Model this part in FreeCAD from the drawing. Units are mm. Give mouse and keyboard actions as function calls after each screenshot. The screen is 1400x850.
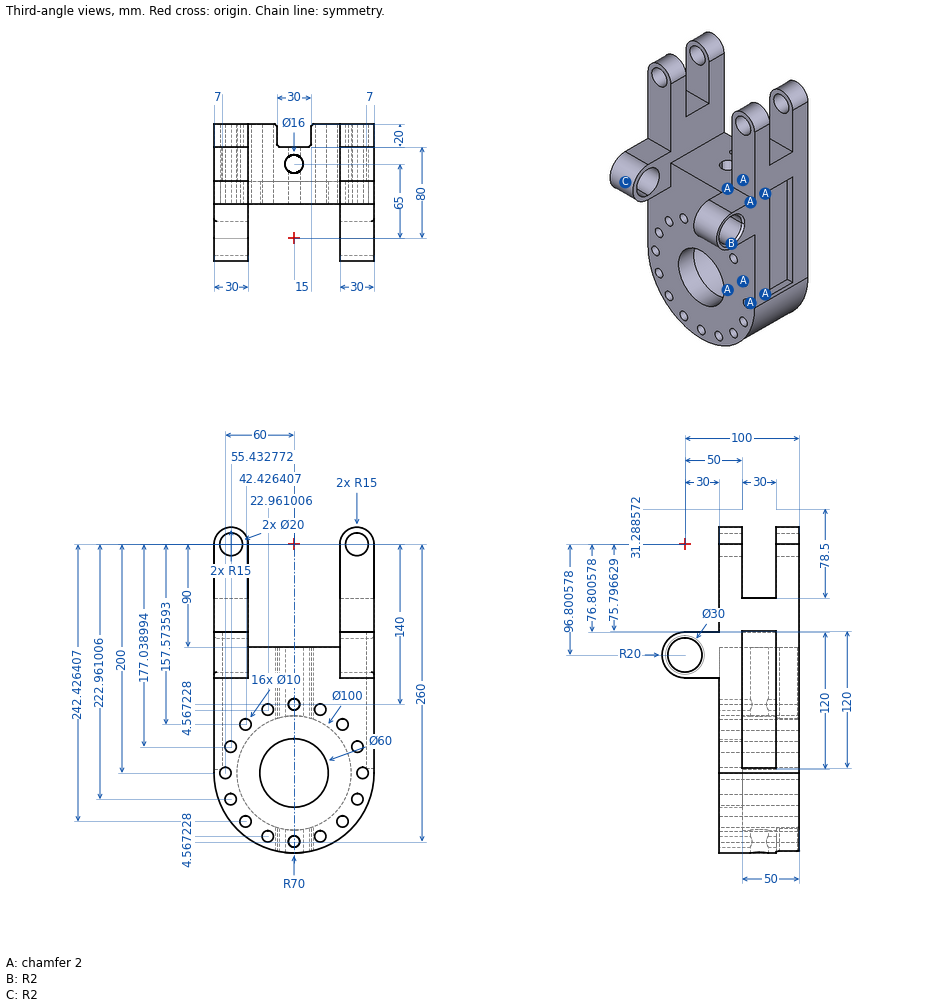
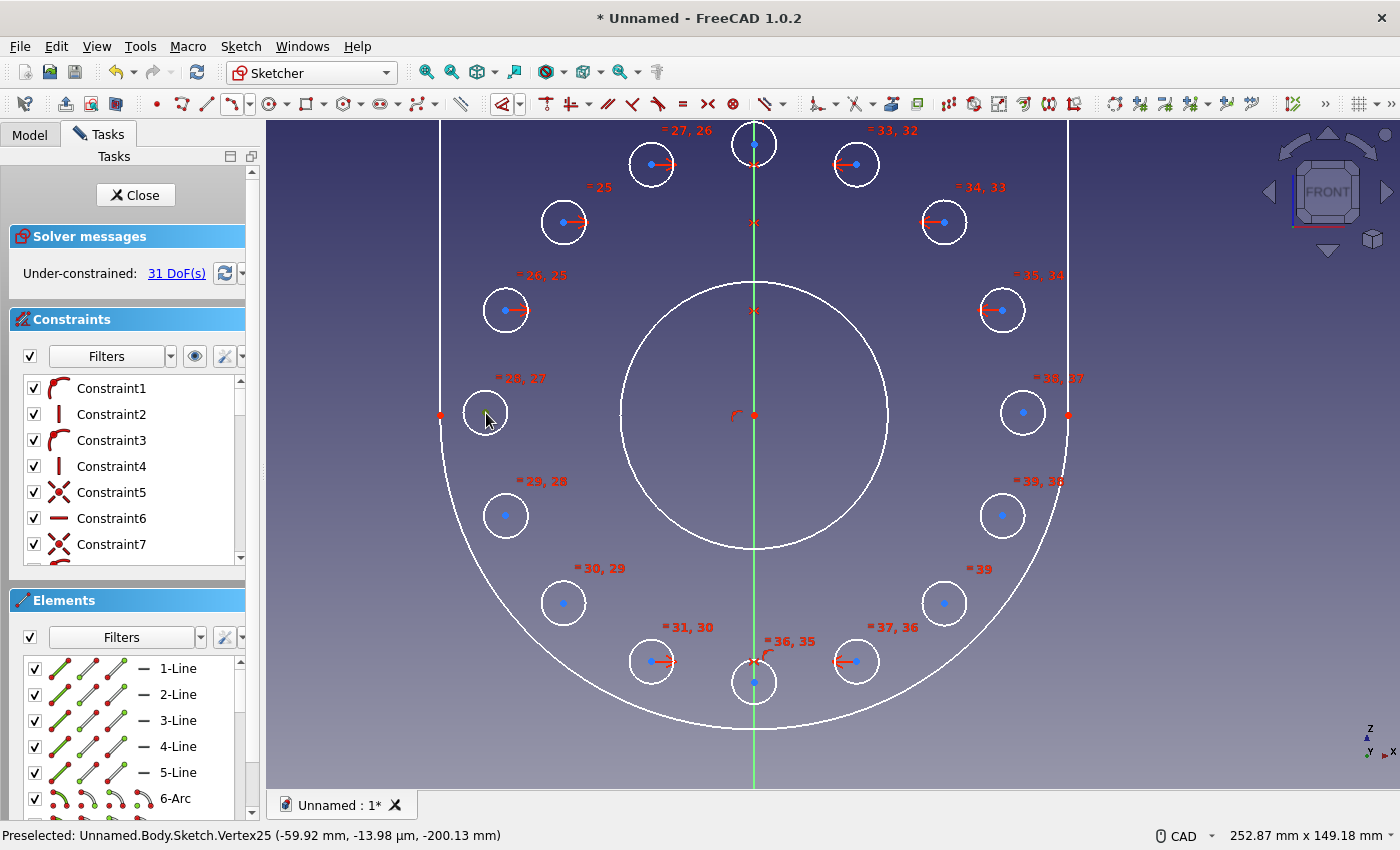
click(1023, 413)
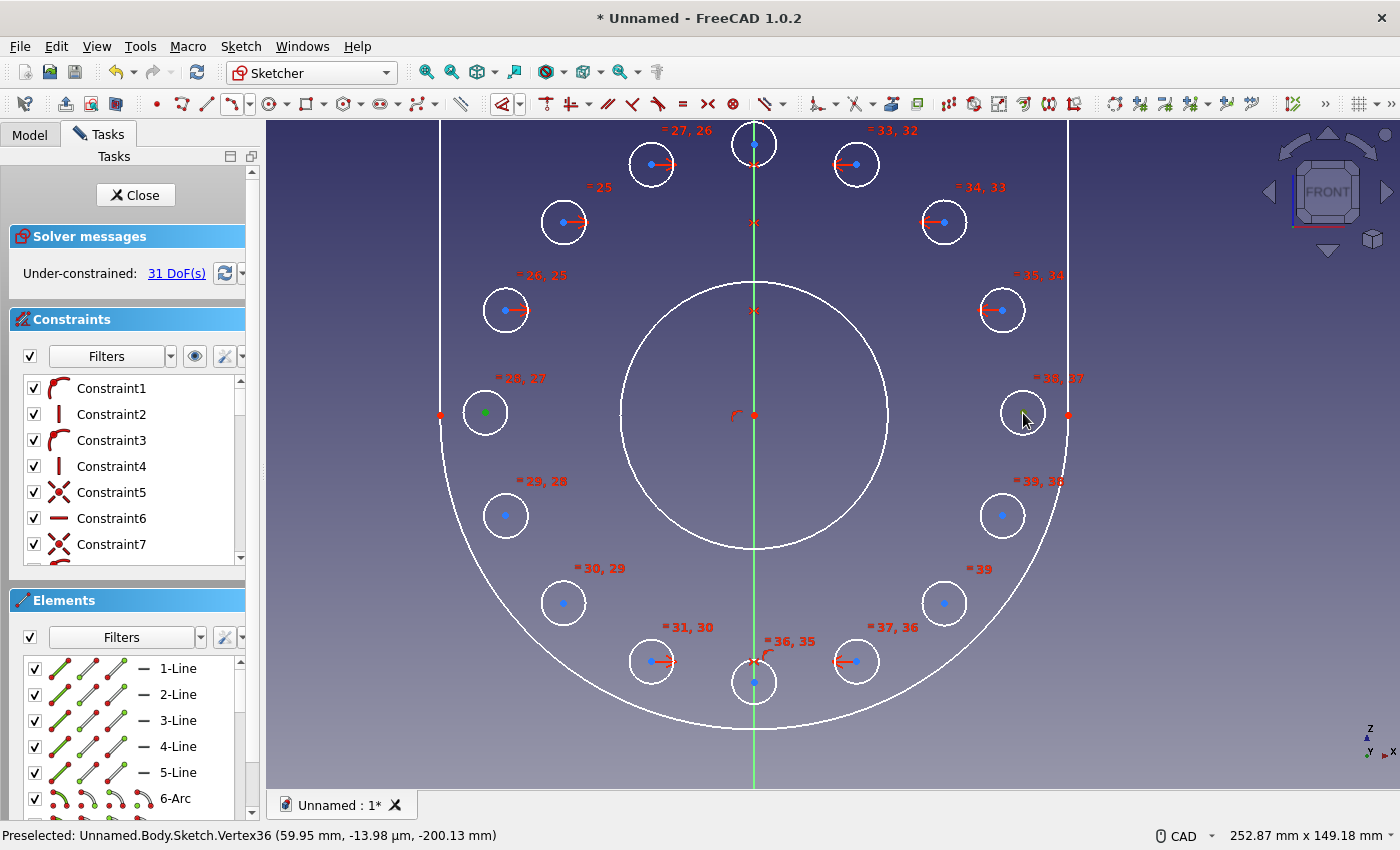
click(754, 630)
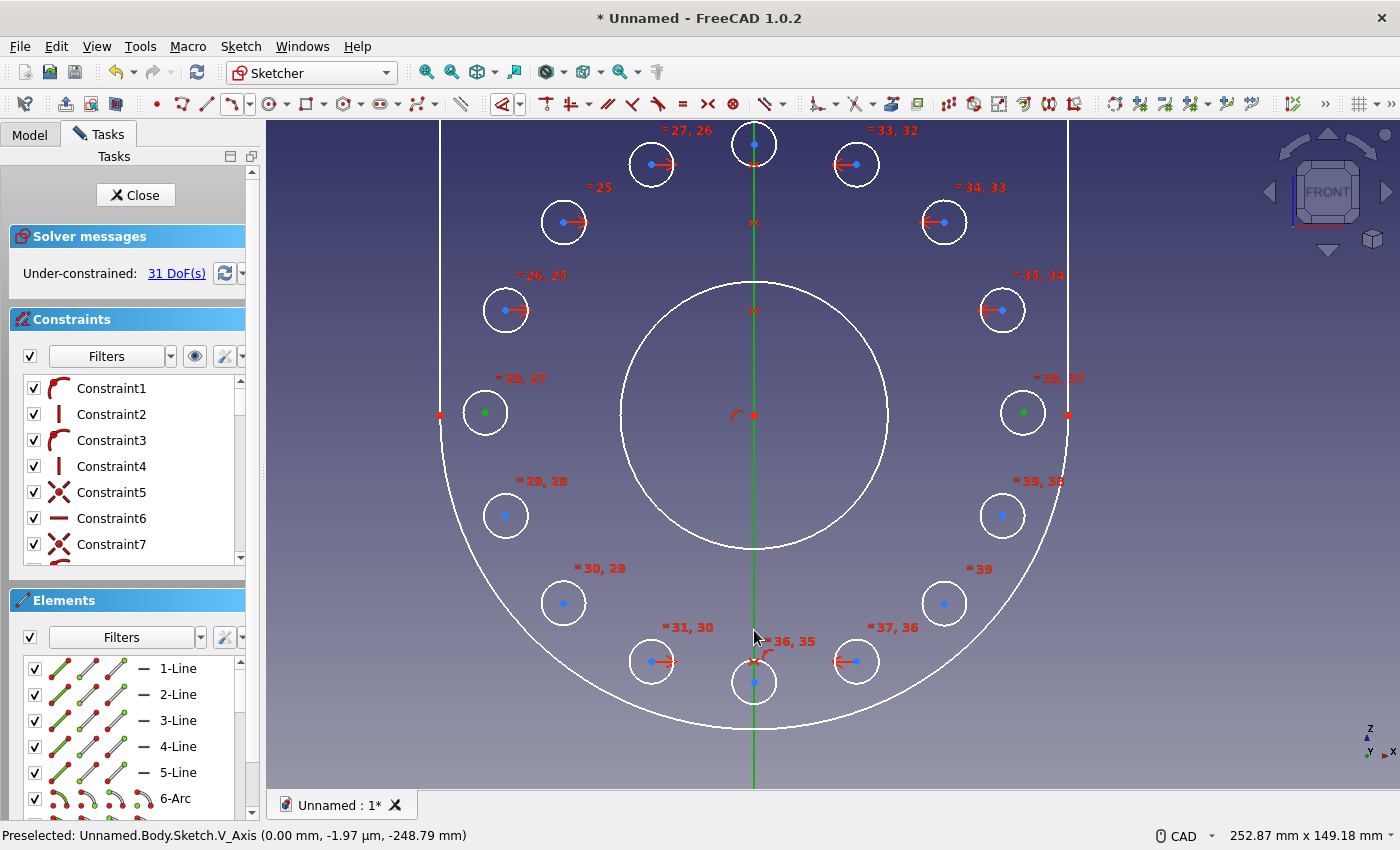
click(708, 104)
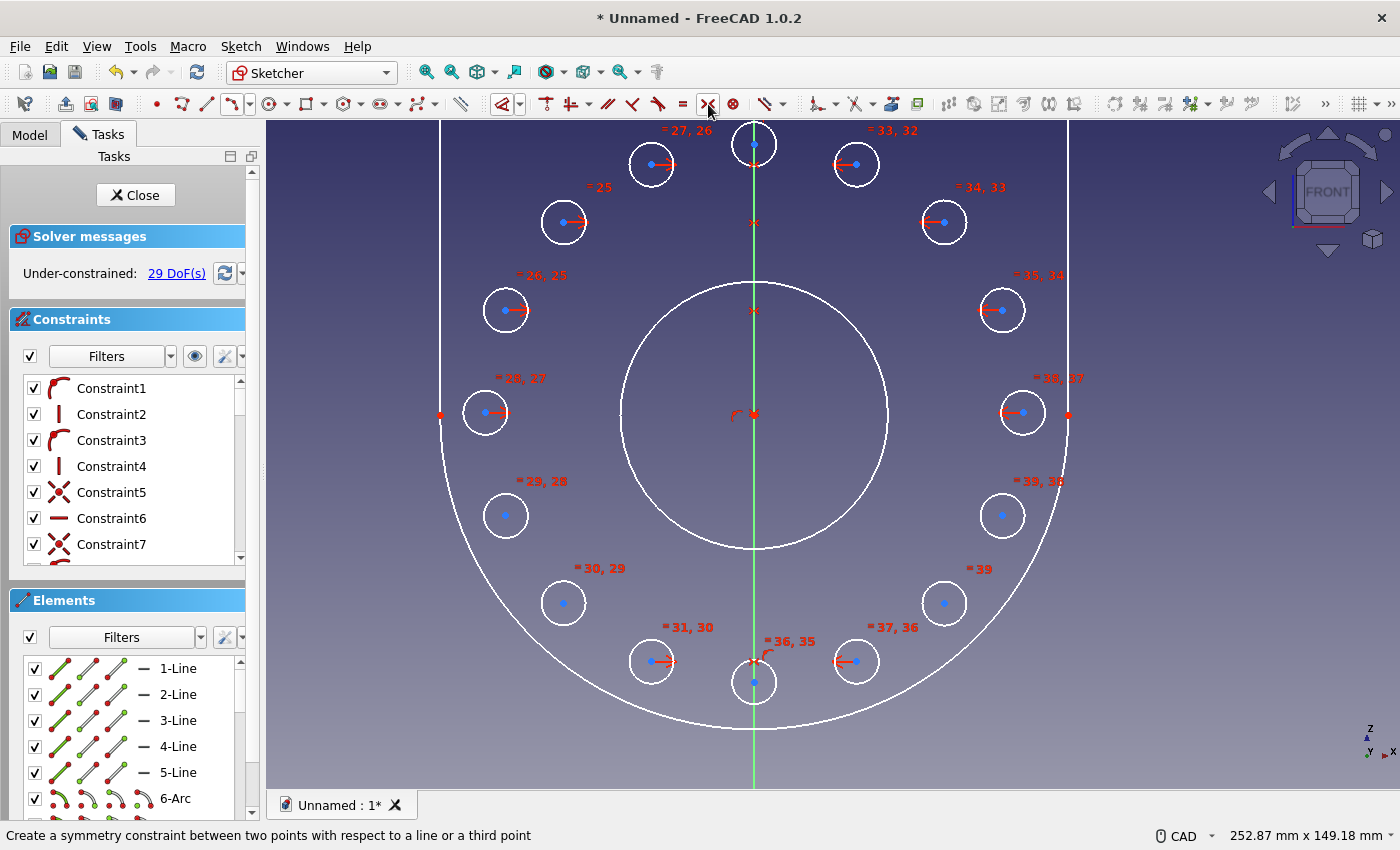
click(506, 516)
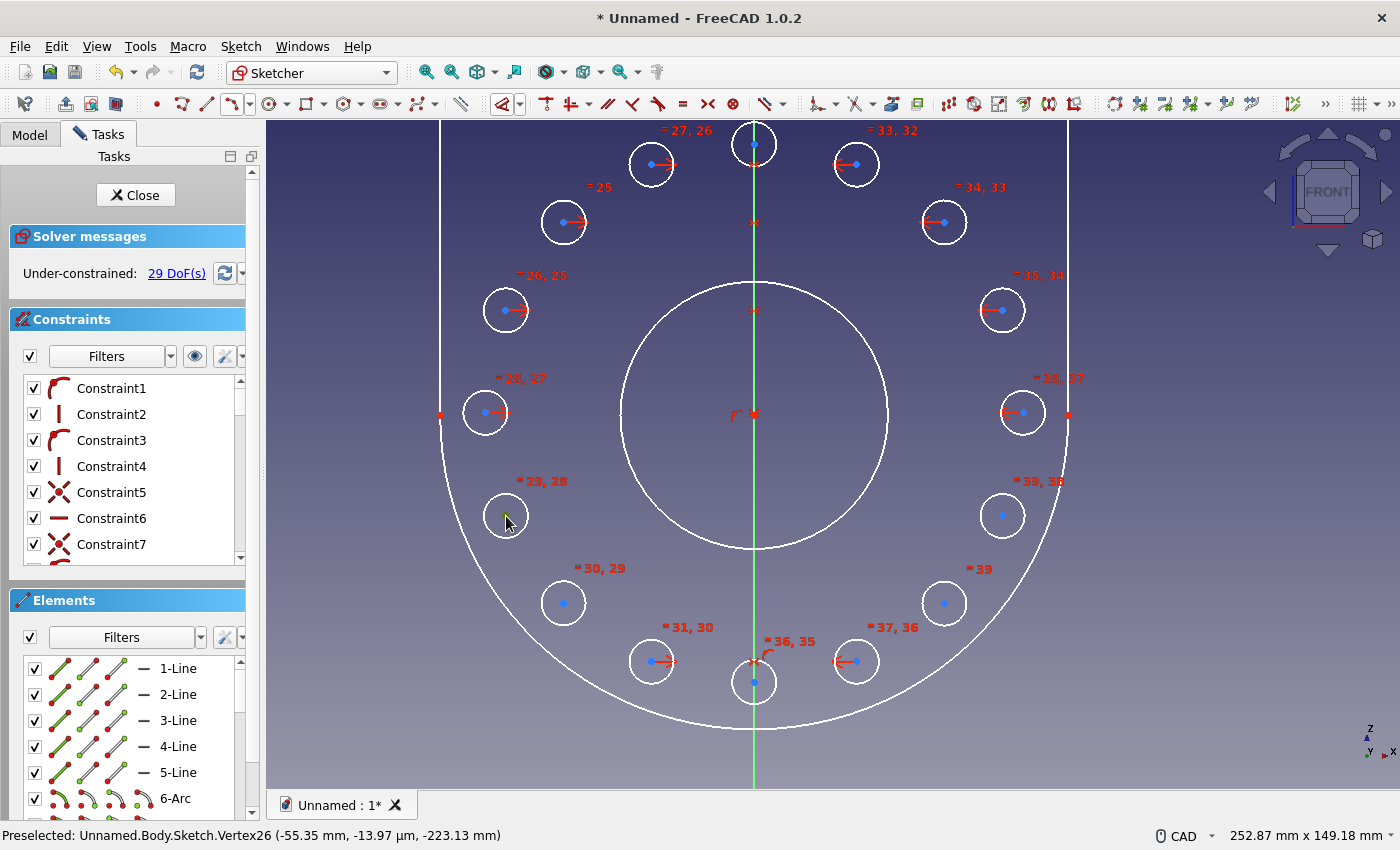
click(1003, 516)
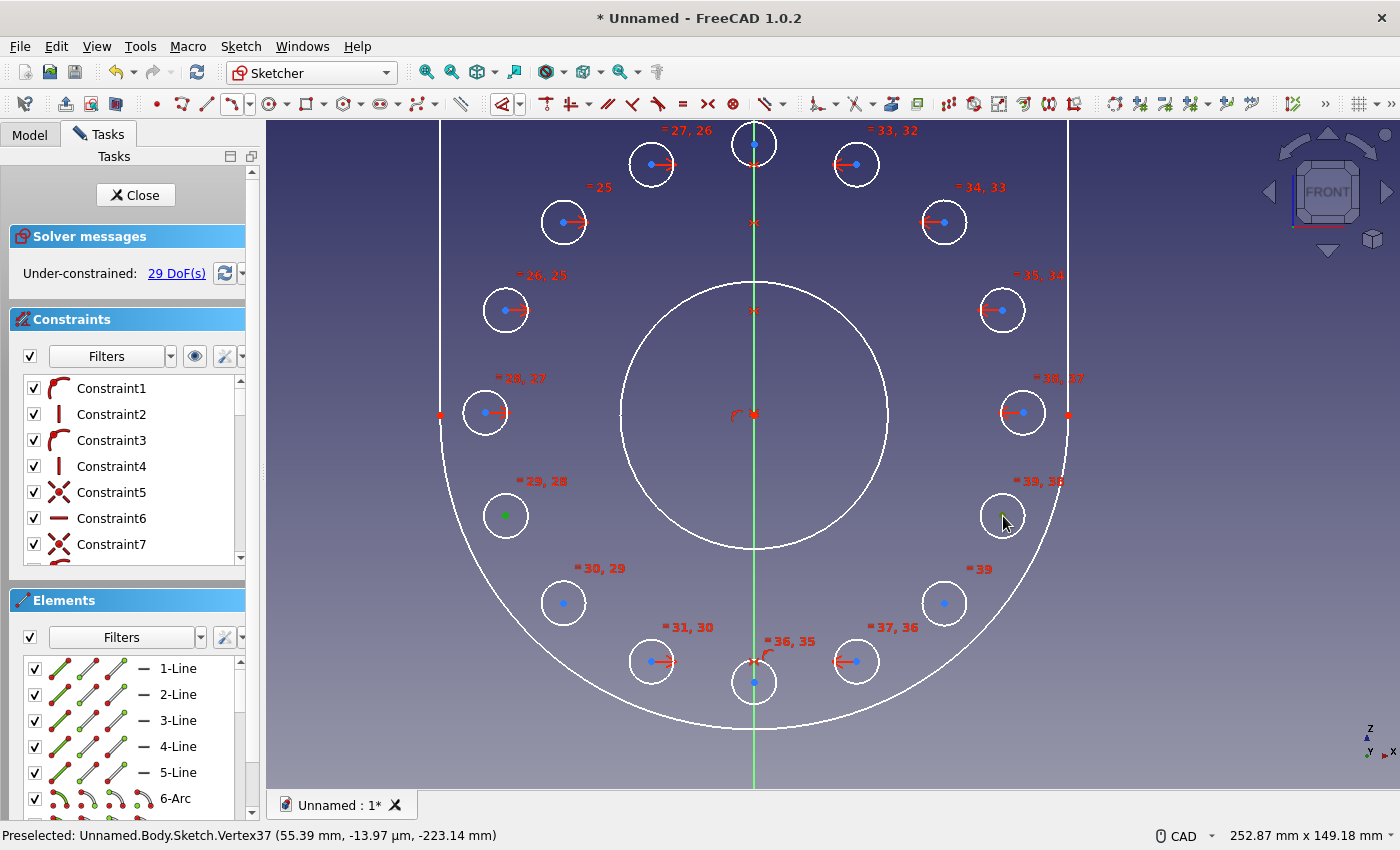
click(754, 630)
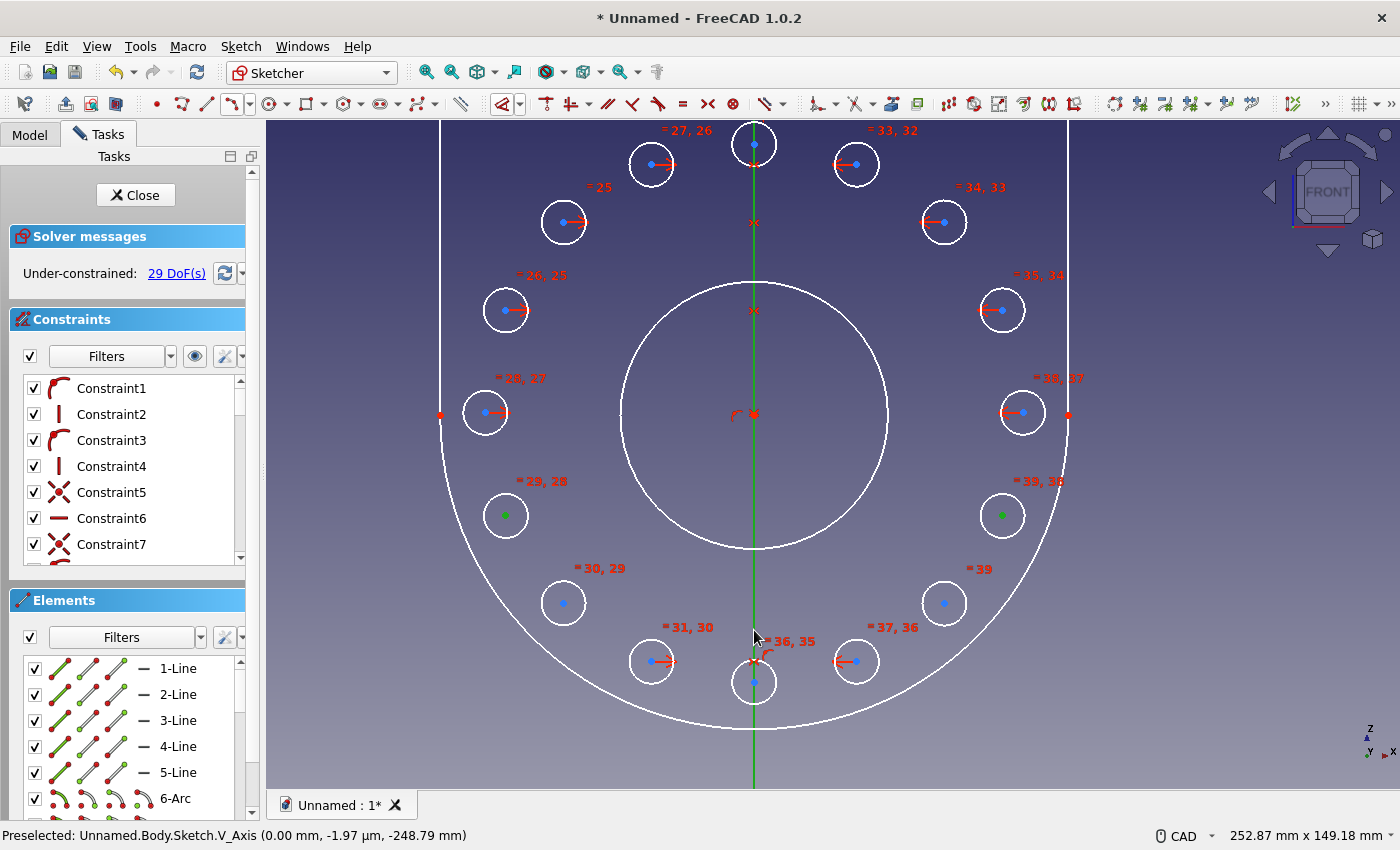
key(s)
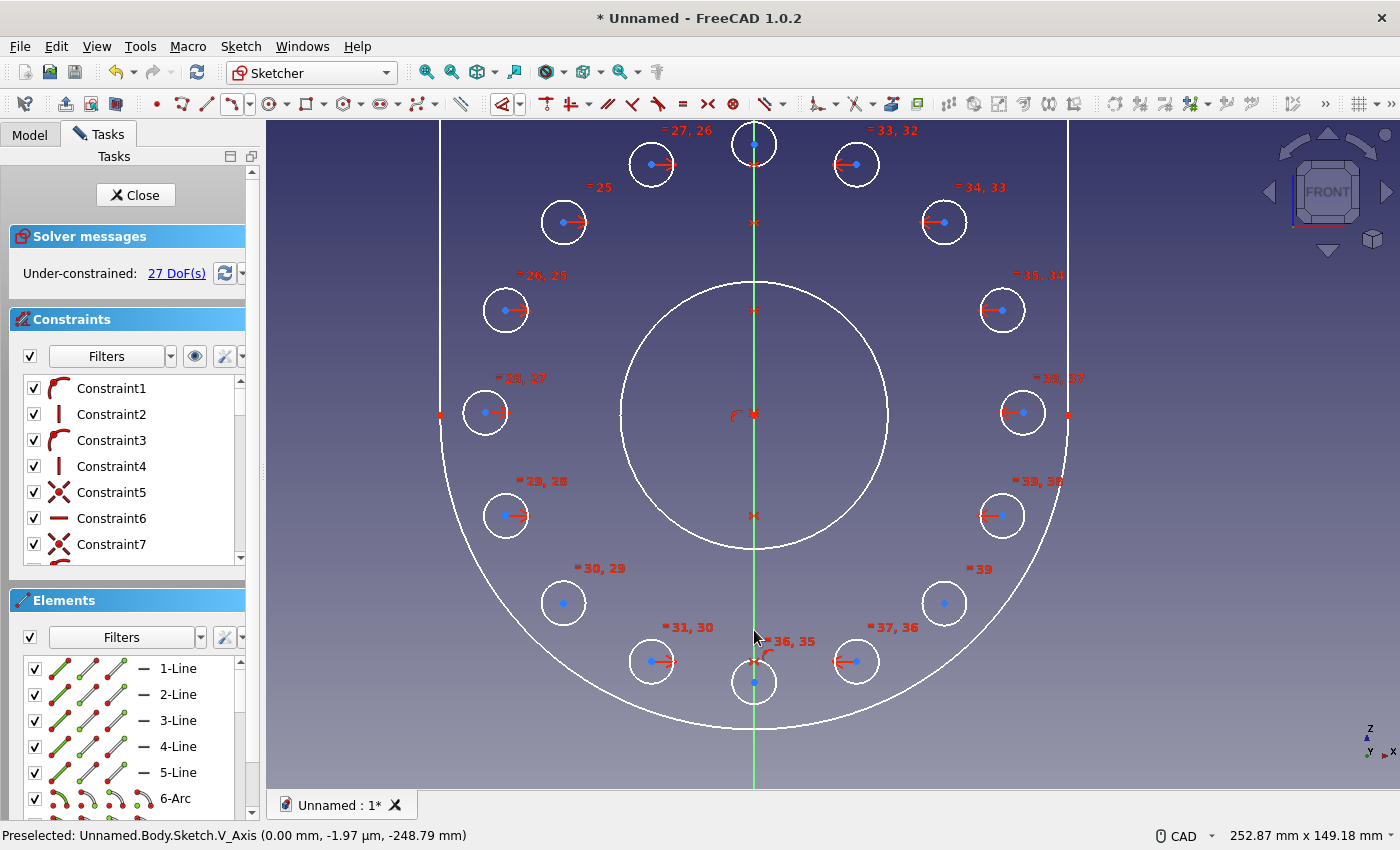
click(564, 603)